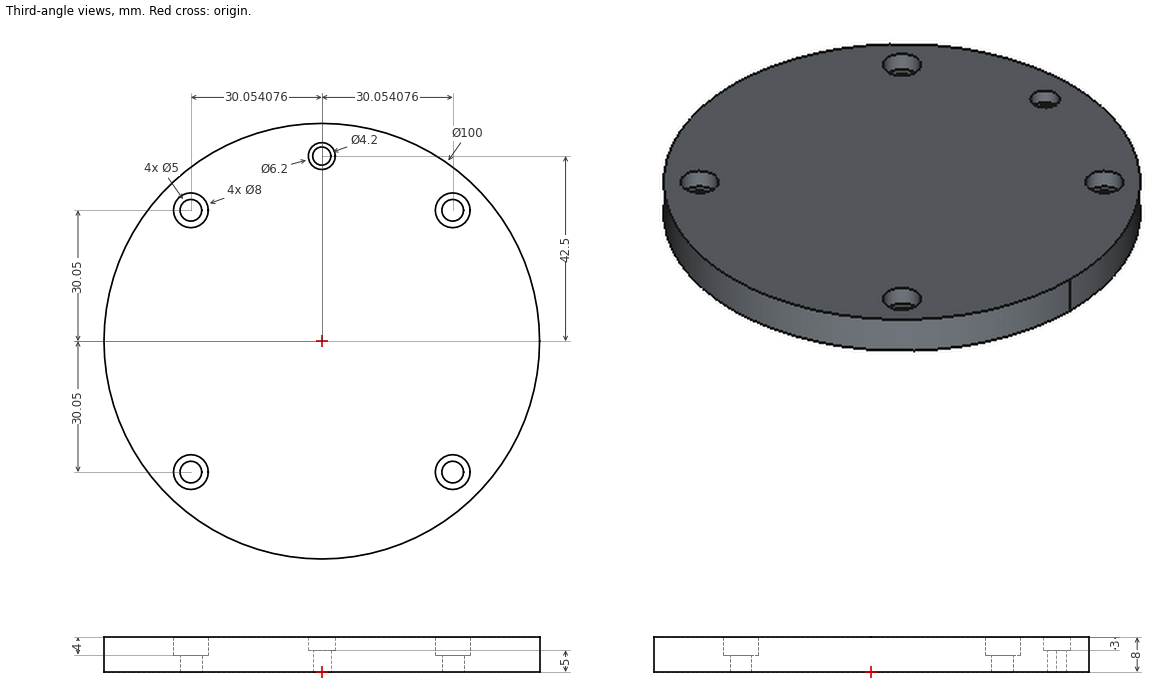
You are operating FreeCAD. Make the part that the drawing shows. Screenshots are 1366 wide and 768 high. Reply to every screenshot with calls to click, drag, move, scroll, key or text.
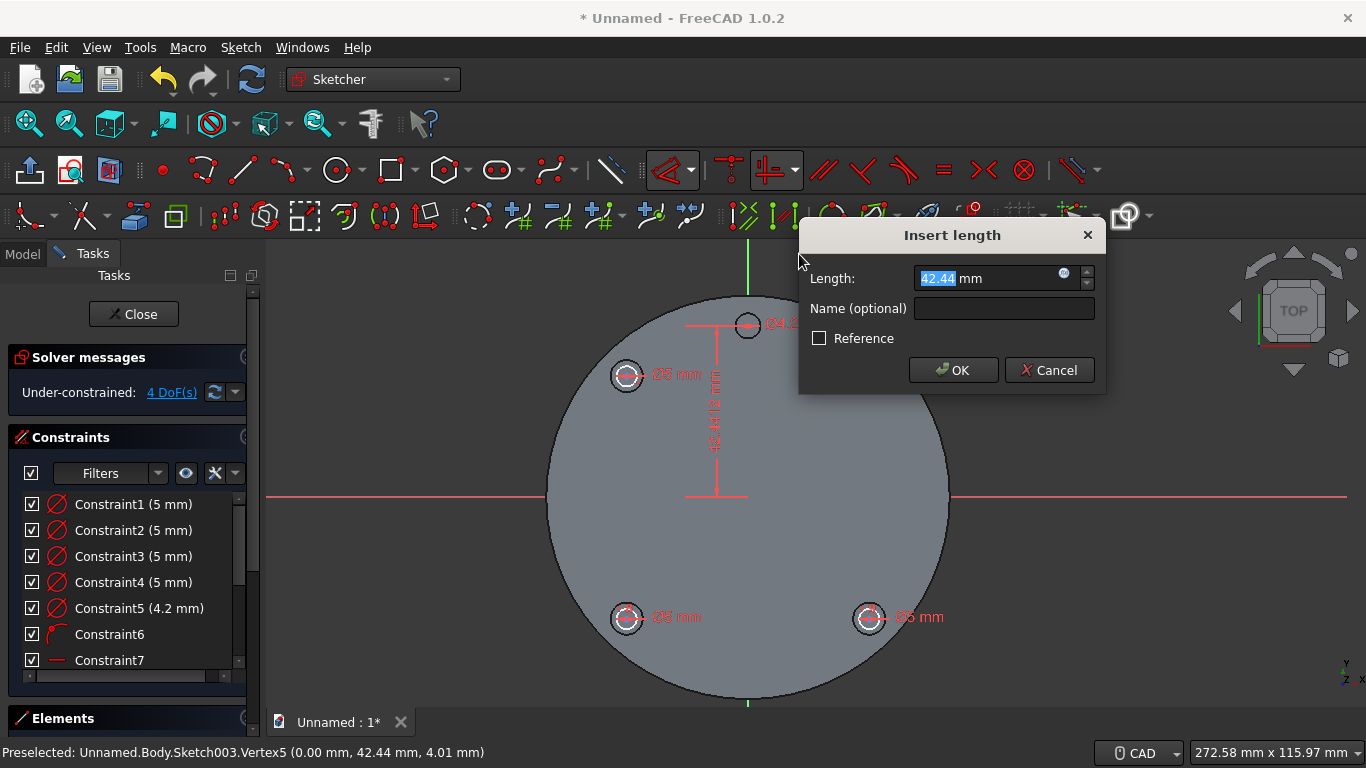
text(42.5)
key(Return)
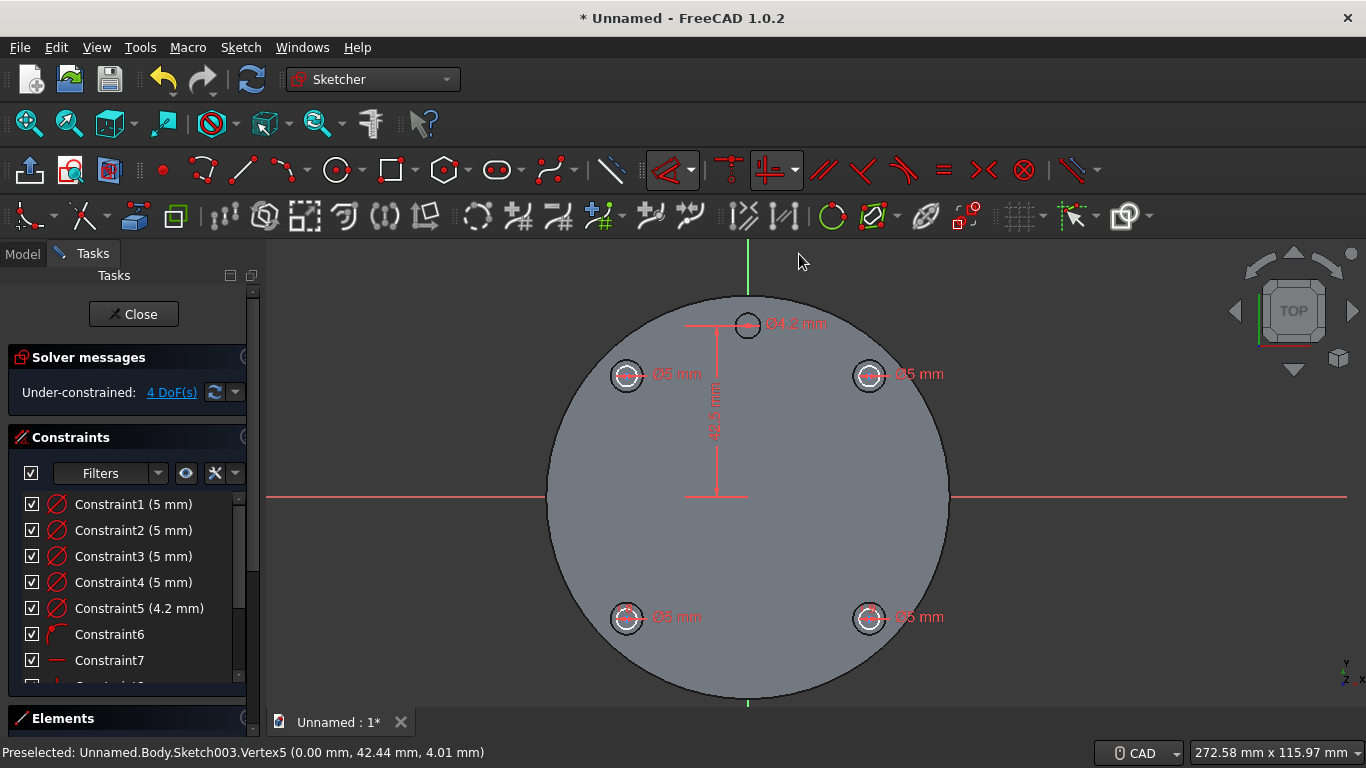
click(627, 376)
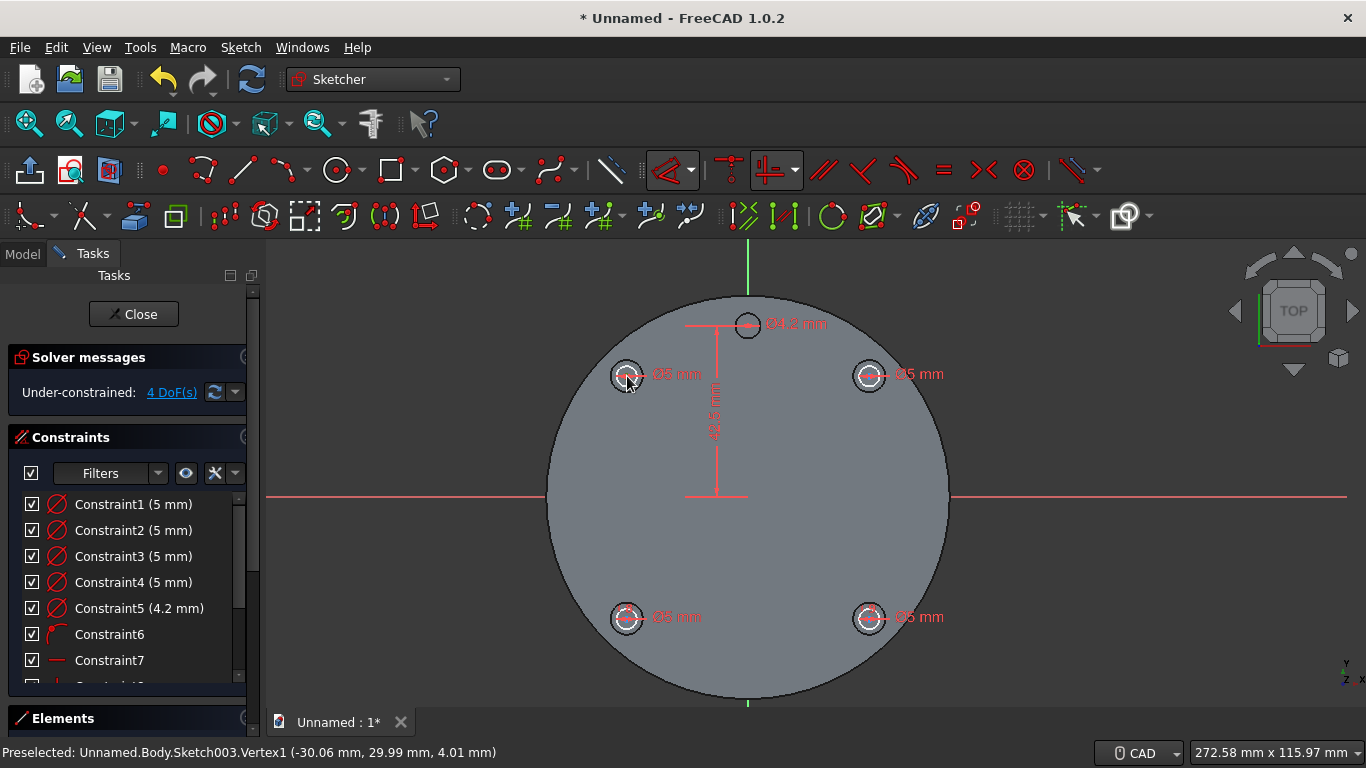
key(i)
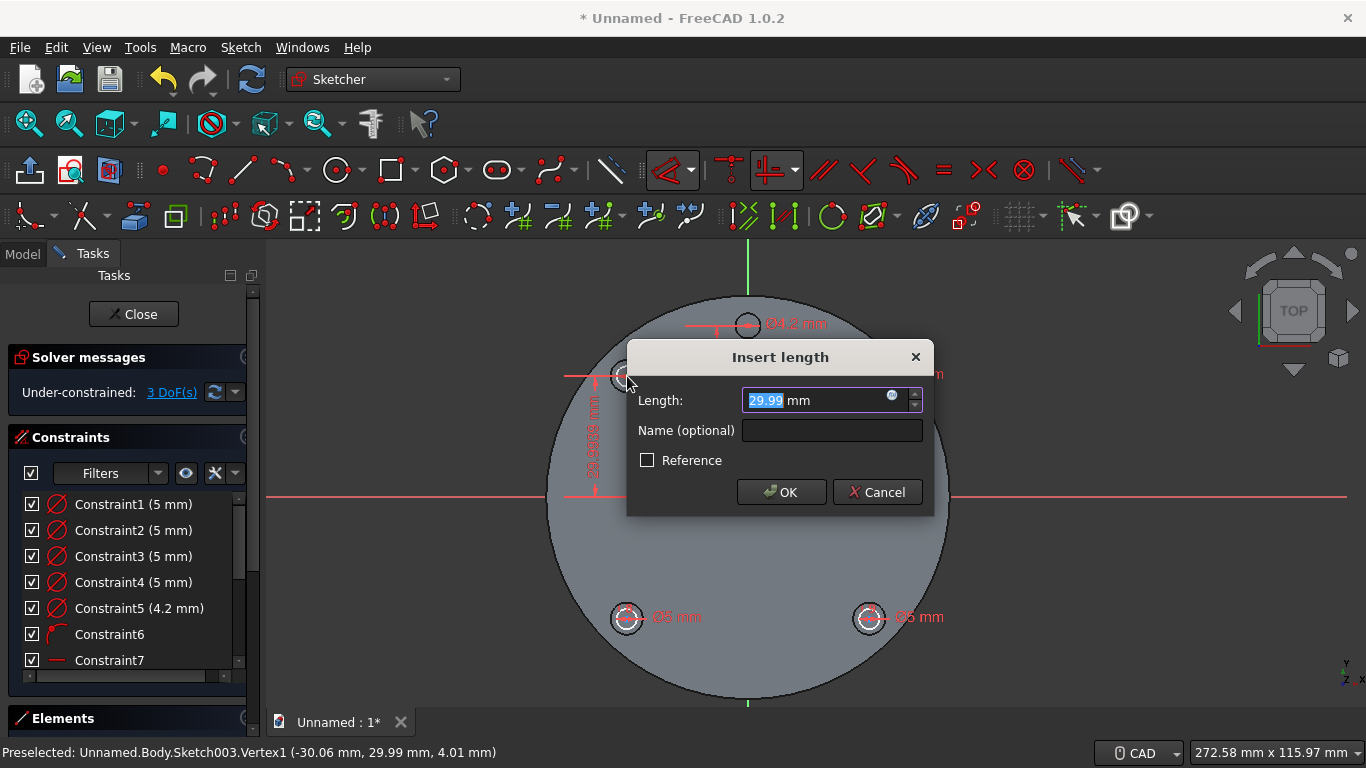
text(30.05)
key(Return)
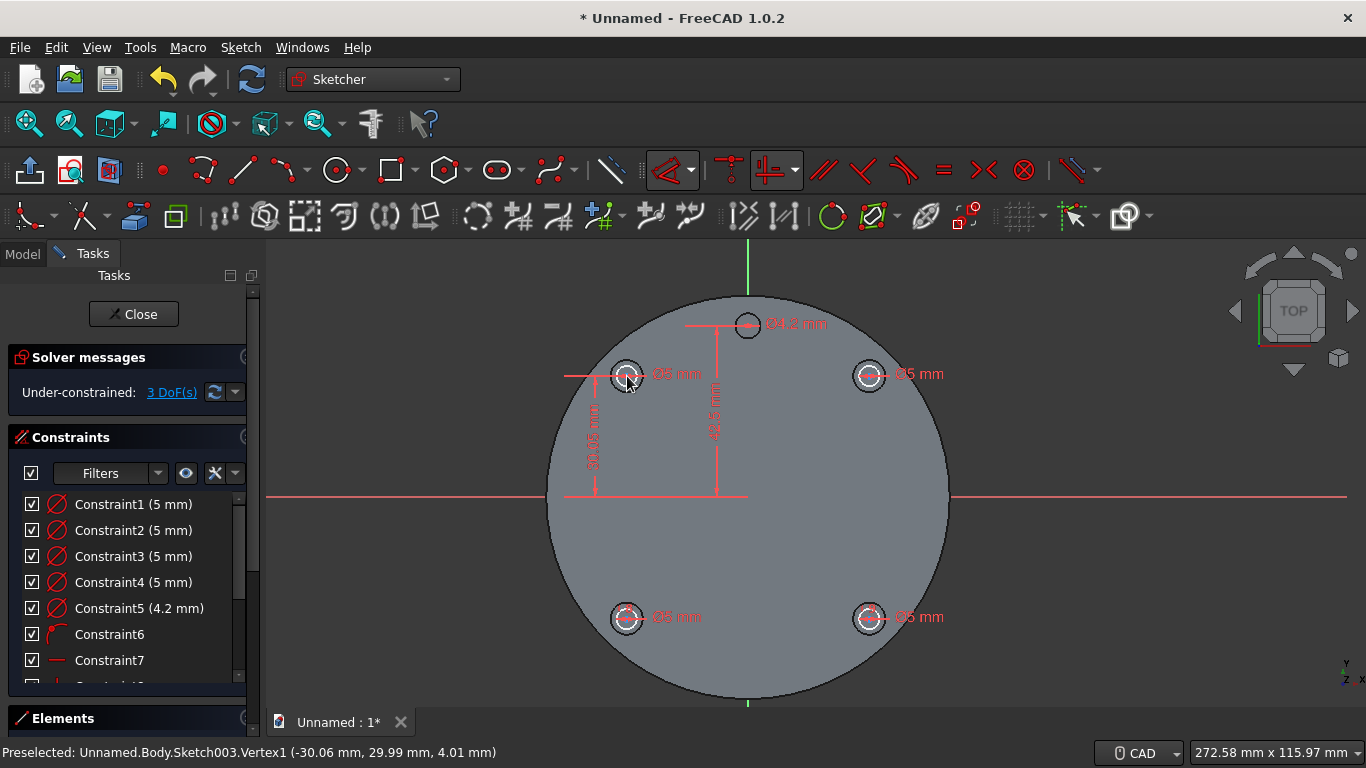
click(627, 619)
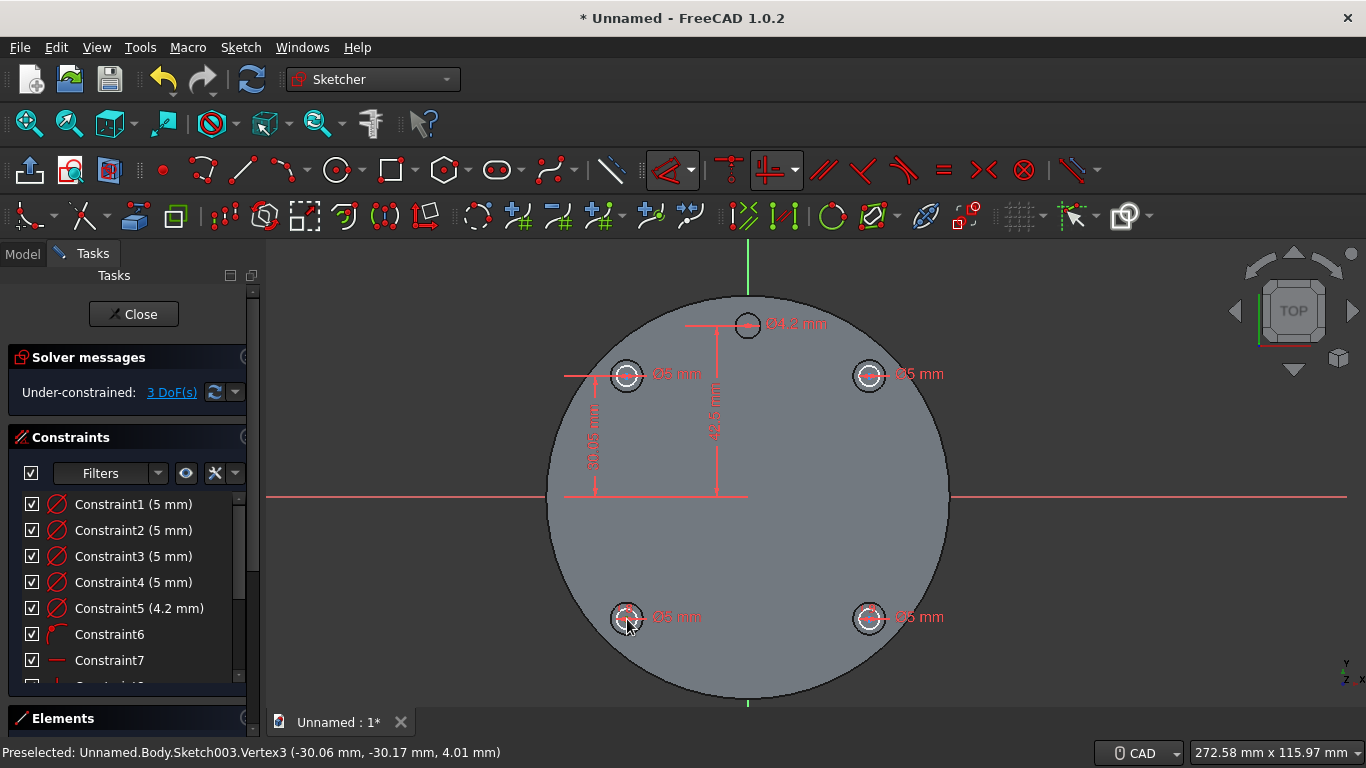
click(694, 170)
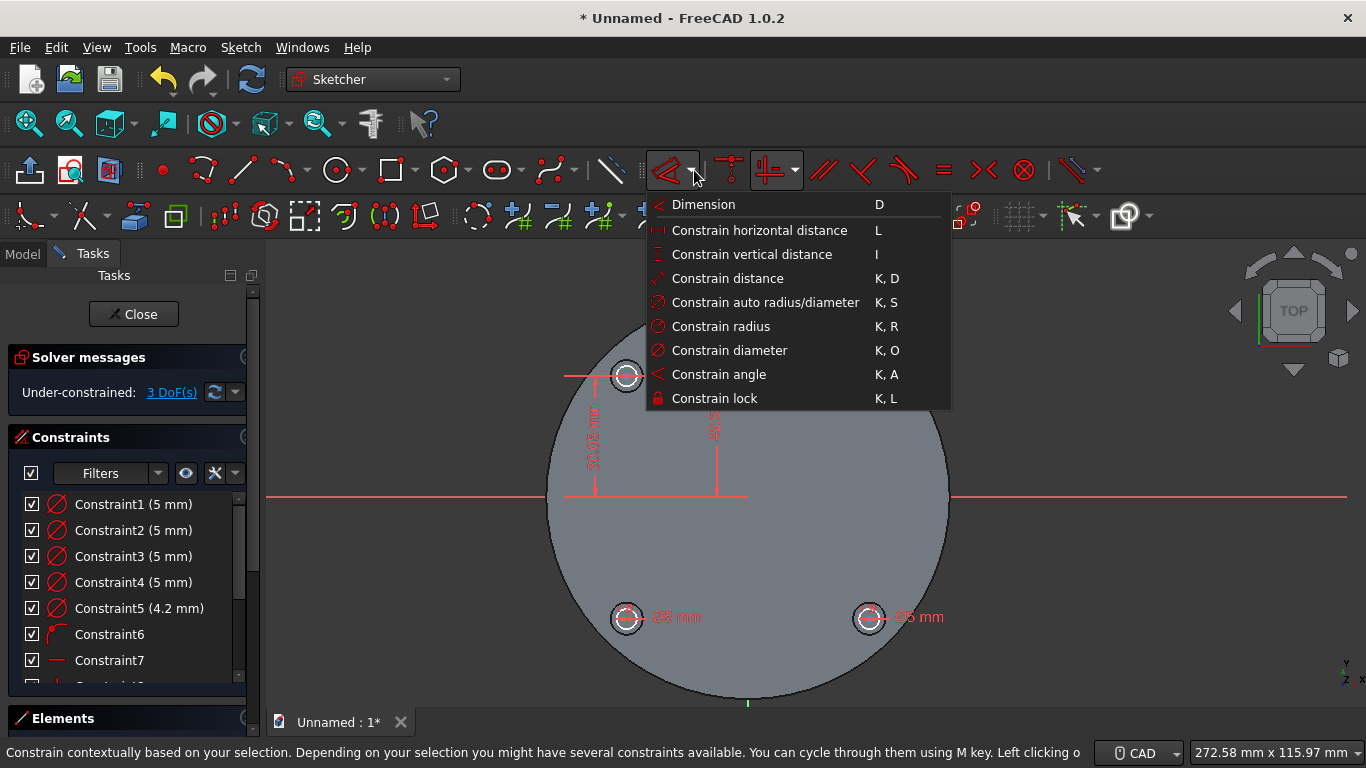
click(799, 254)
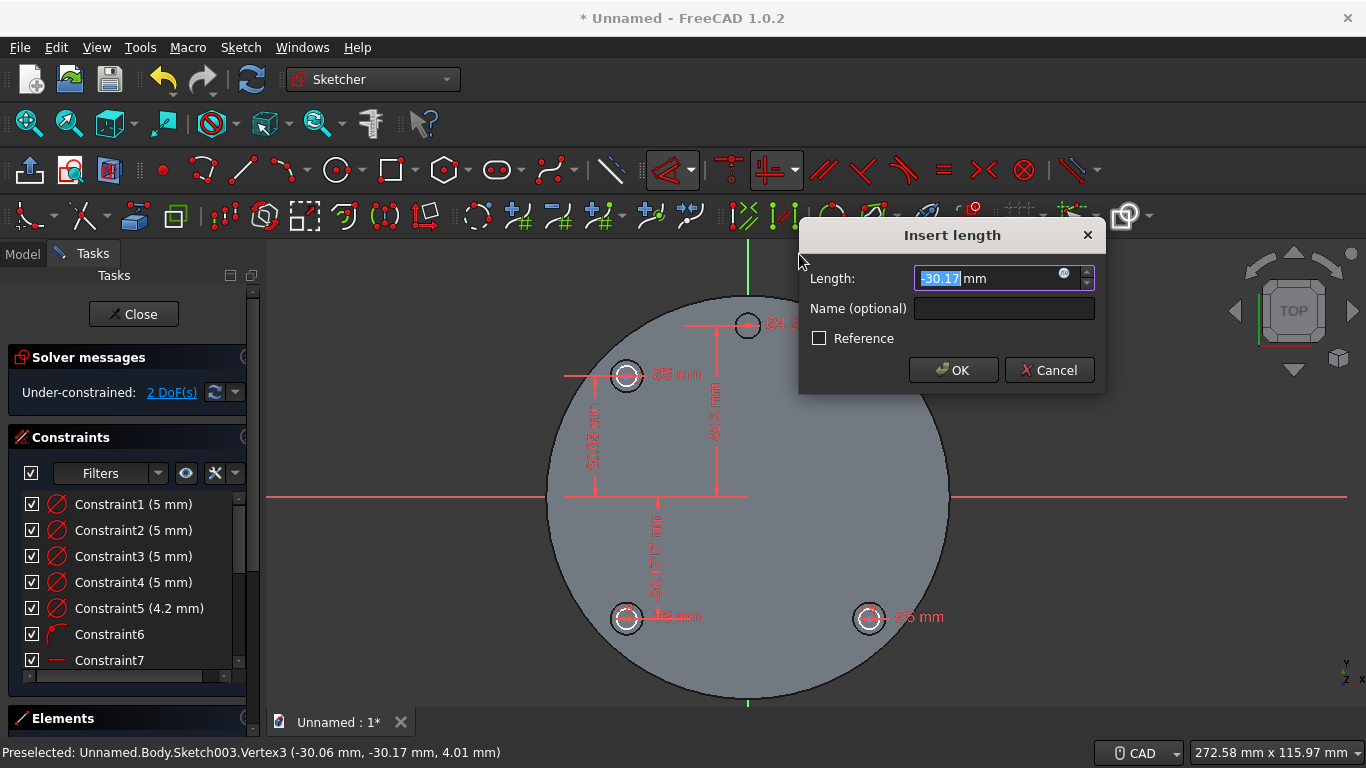
text(-30.05)
key(Return)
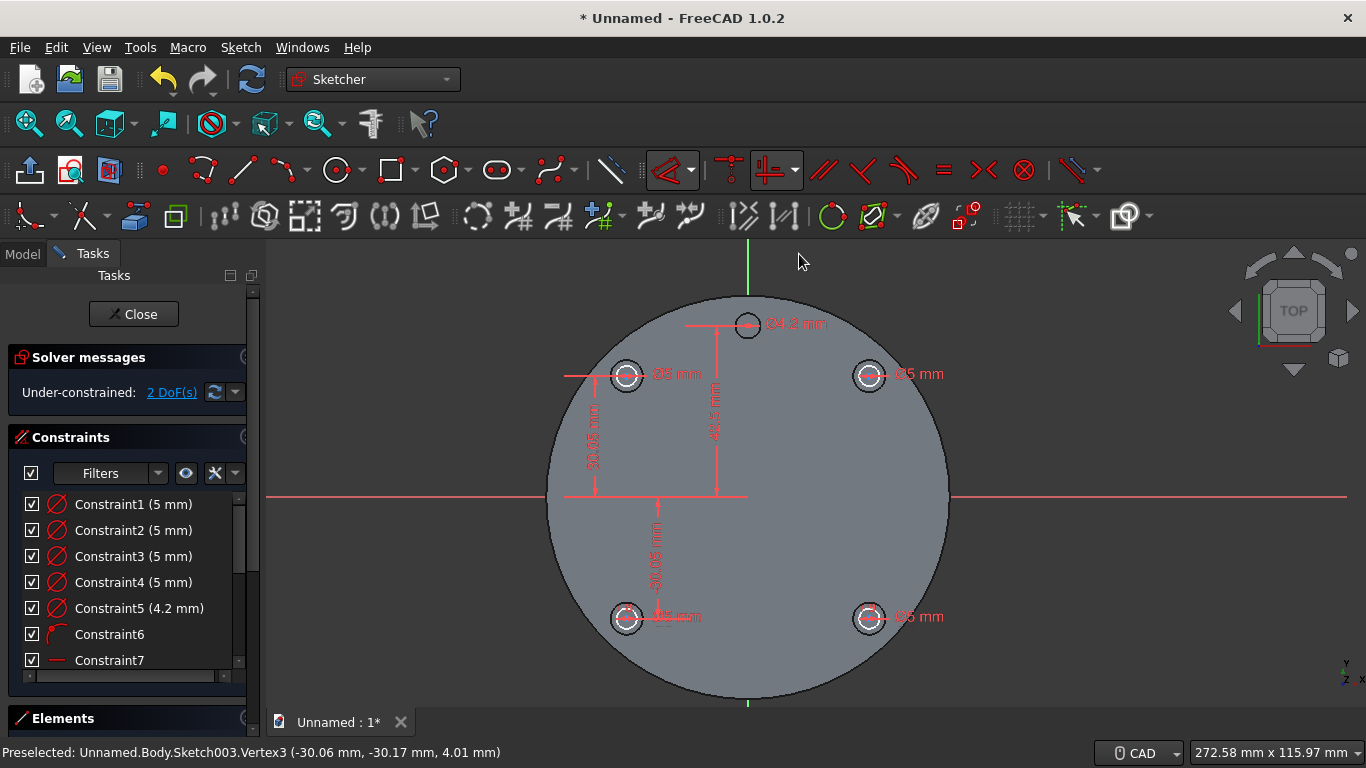
click(627, 376)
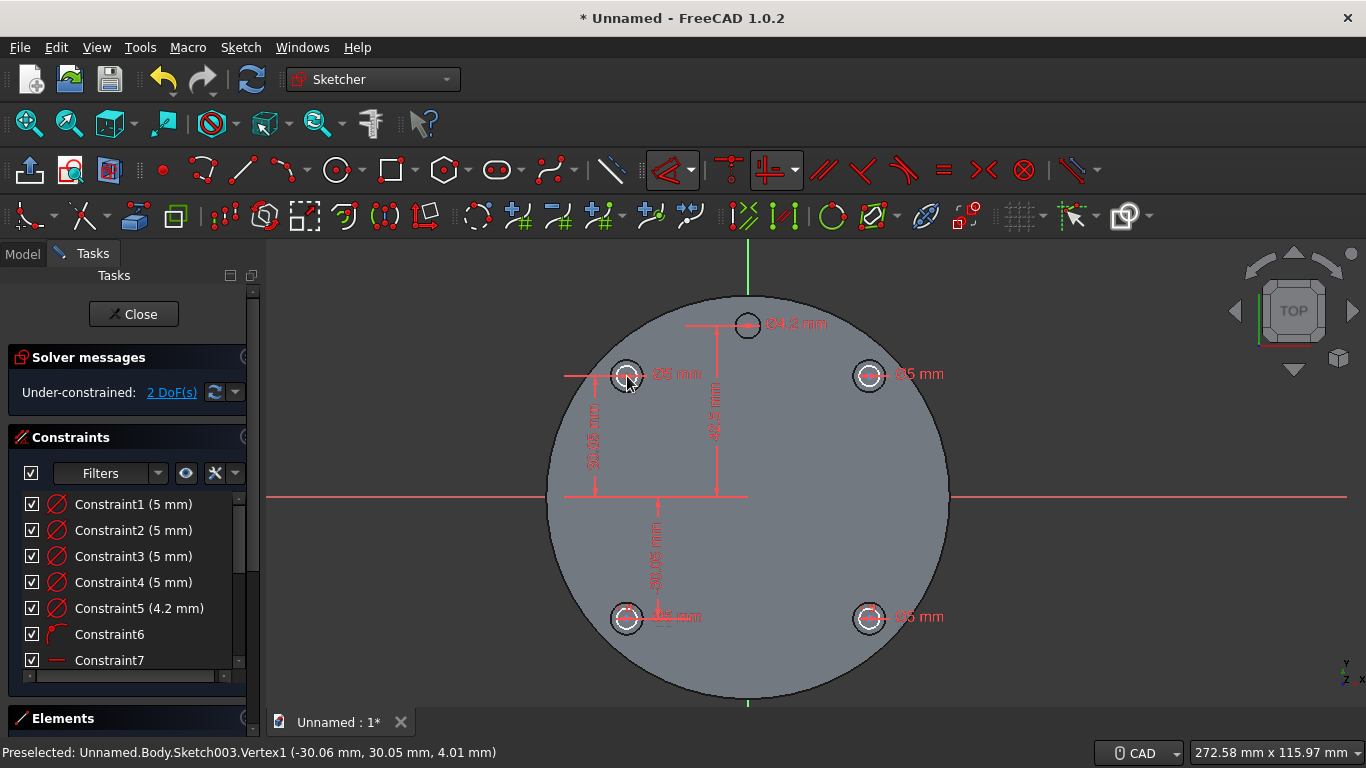
key(l)